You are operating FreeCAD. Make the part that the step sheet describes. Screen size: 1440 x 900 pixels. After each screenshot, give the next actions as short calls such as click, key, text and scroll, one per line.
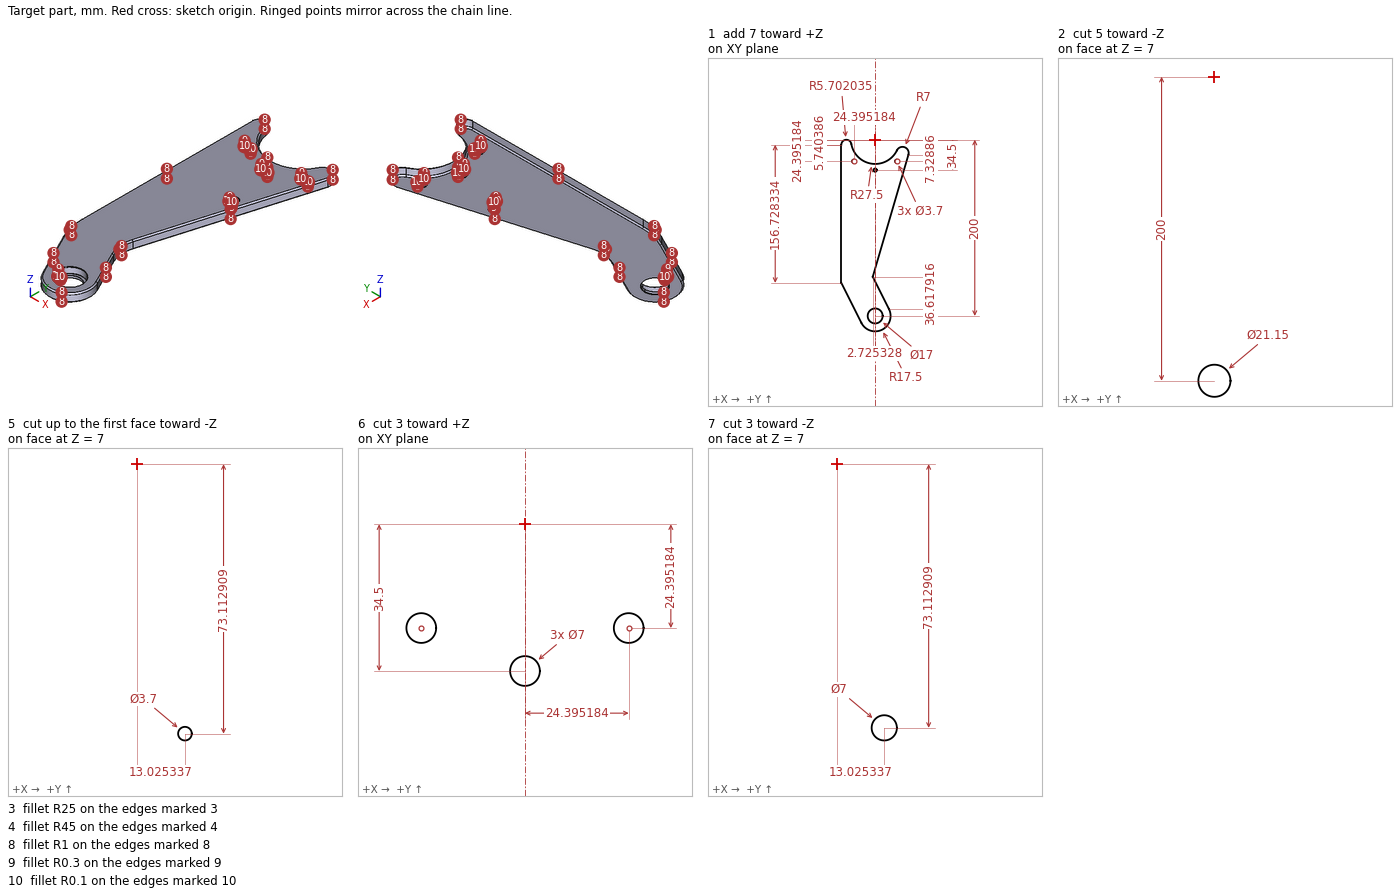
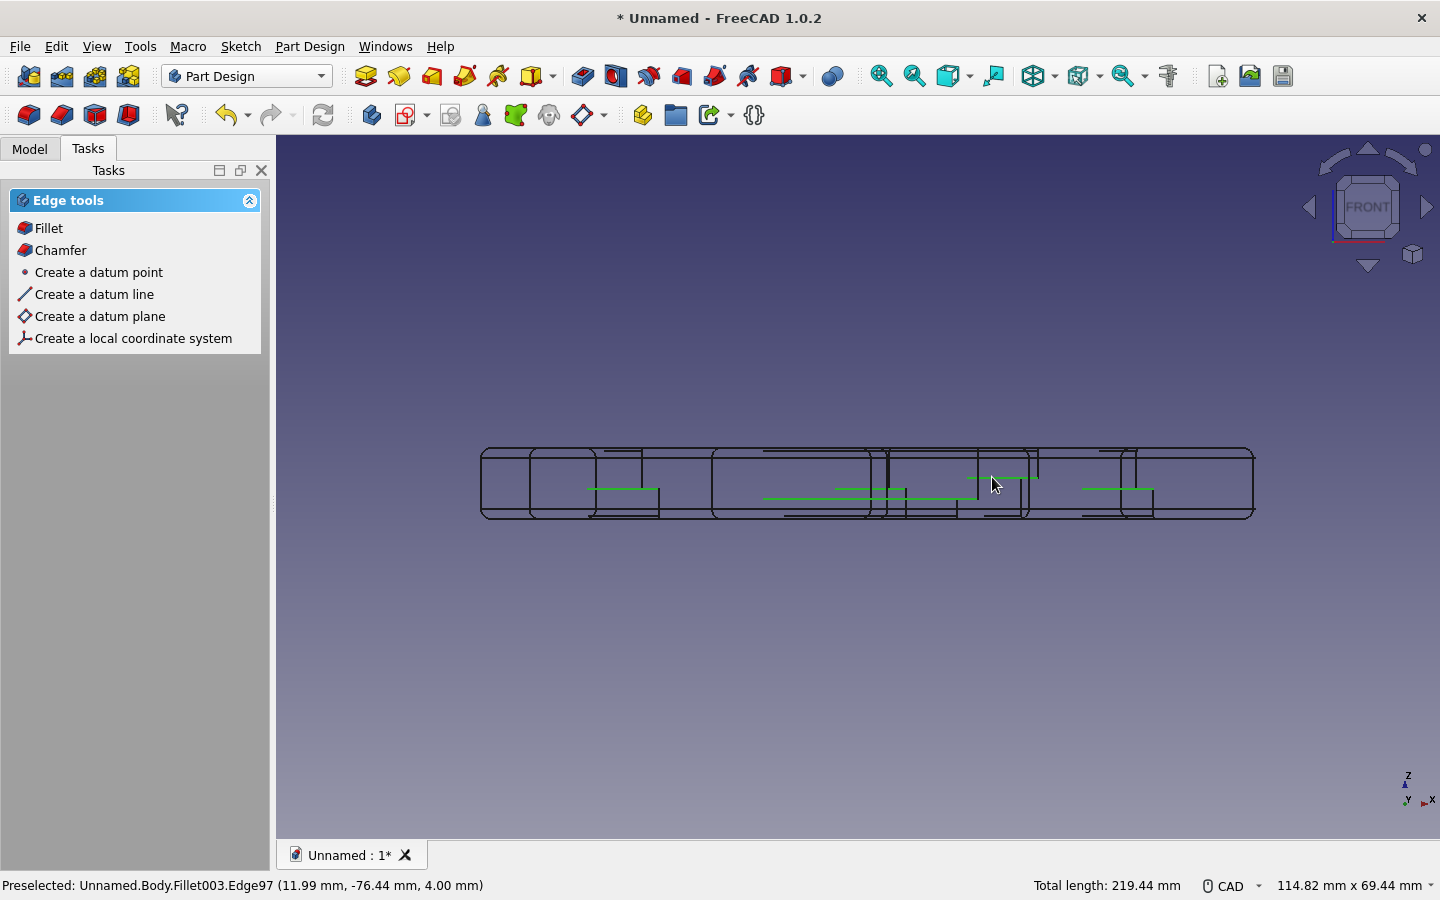
click(882, 76)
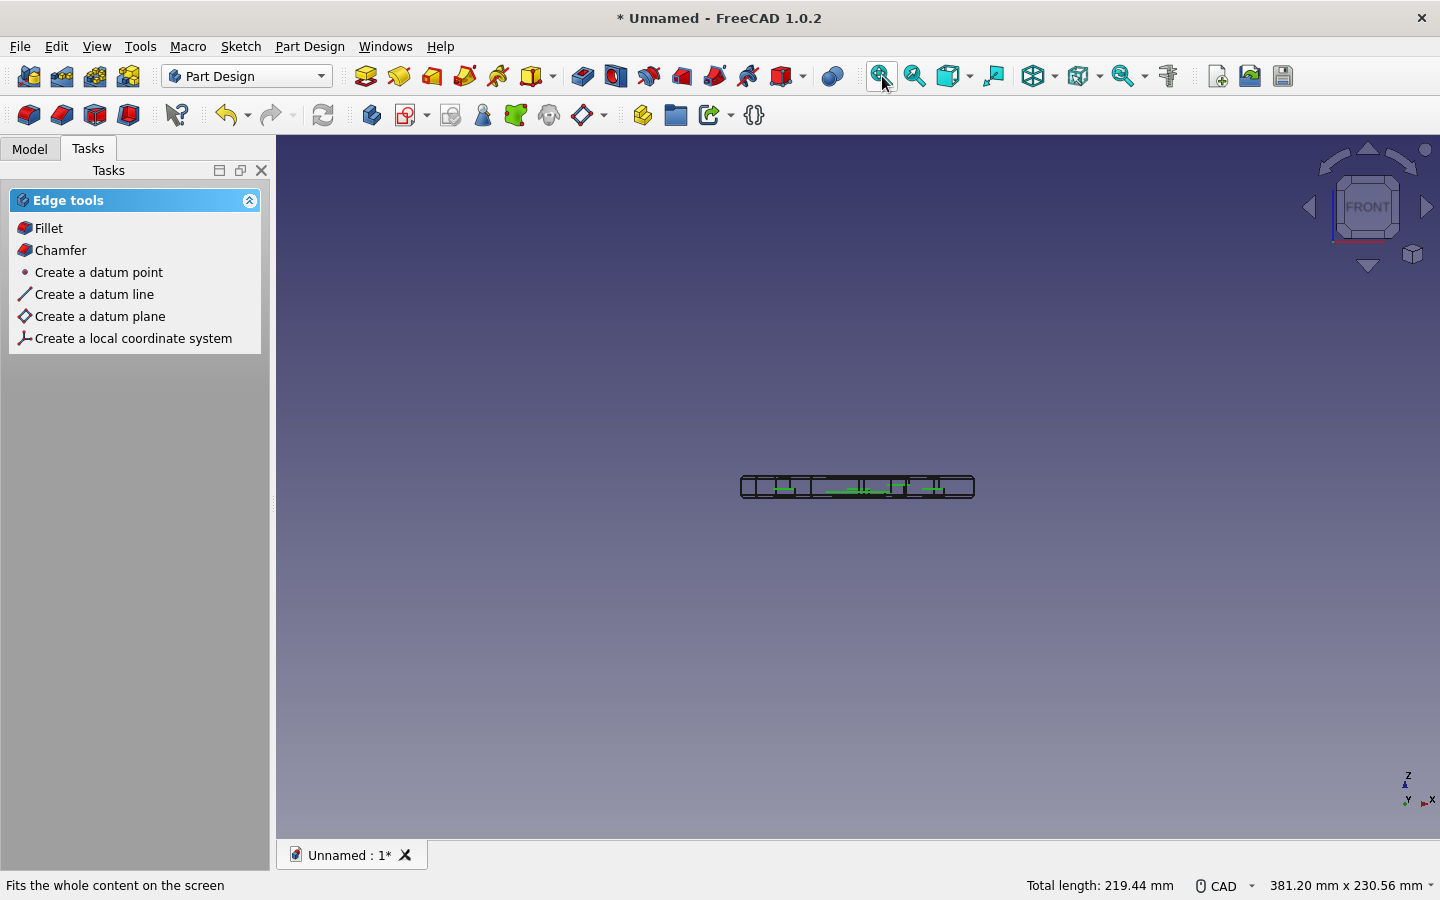
key(3)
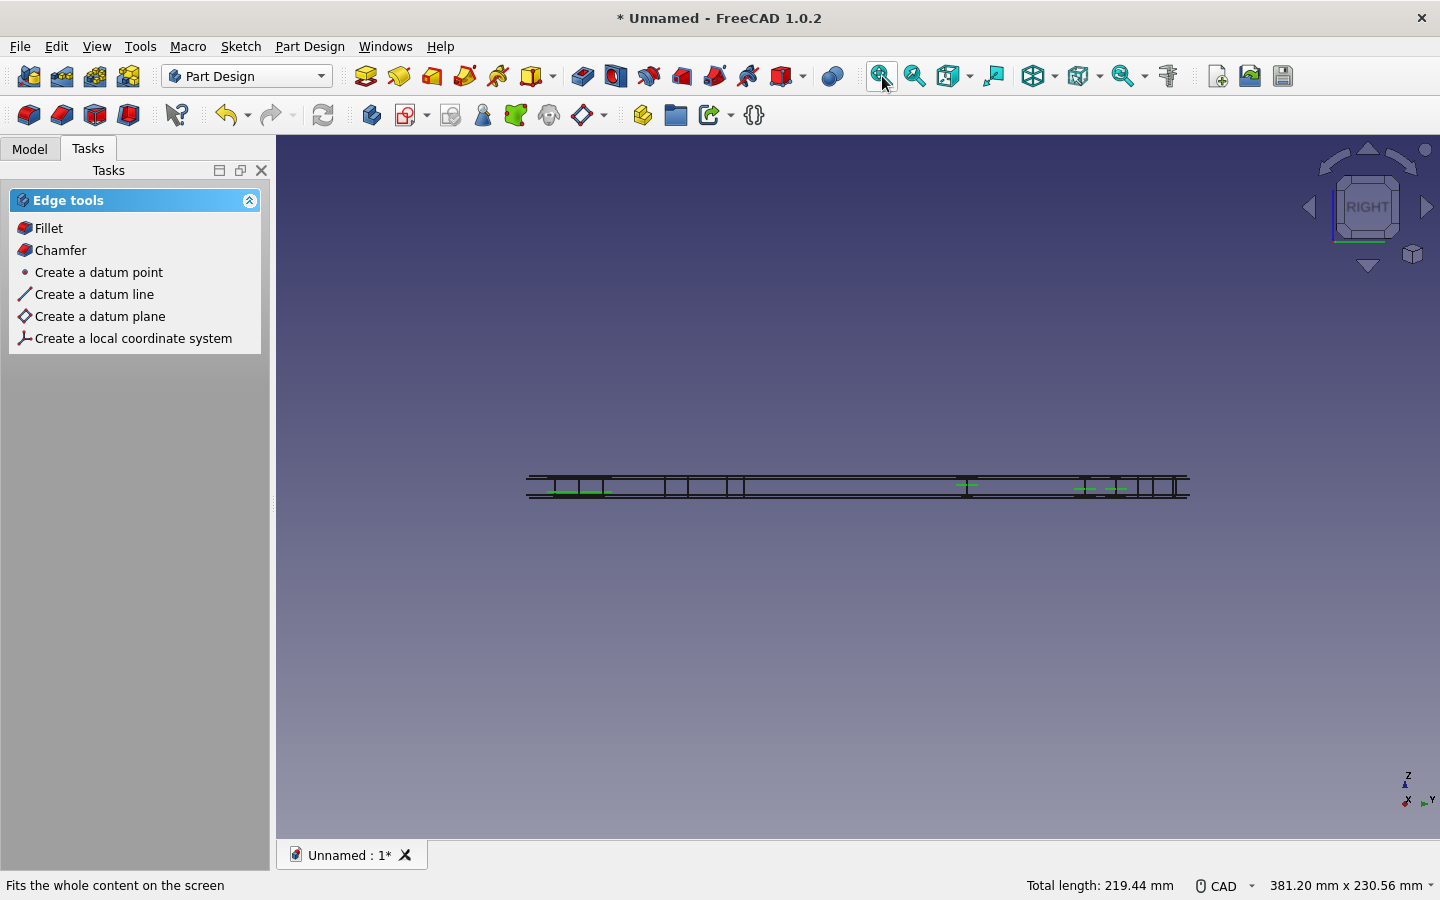
scroll(1085, 488, up, 6)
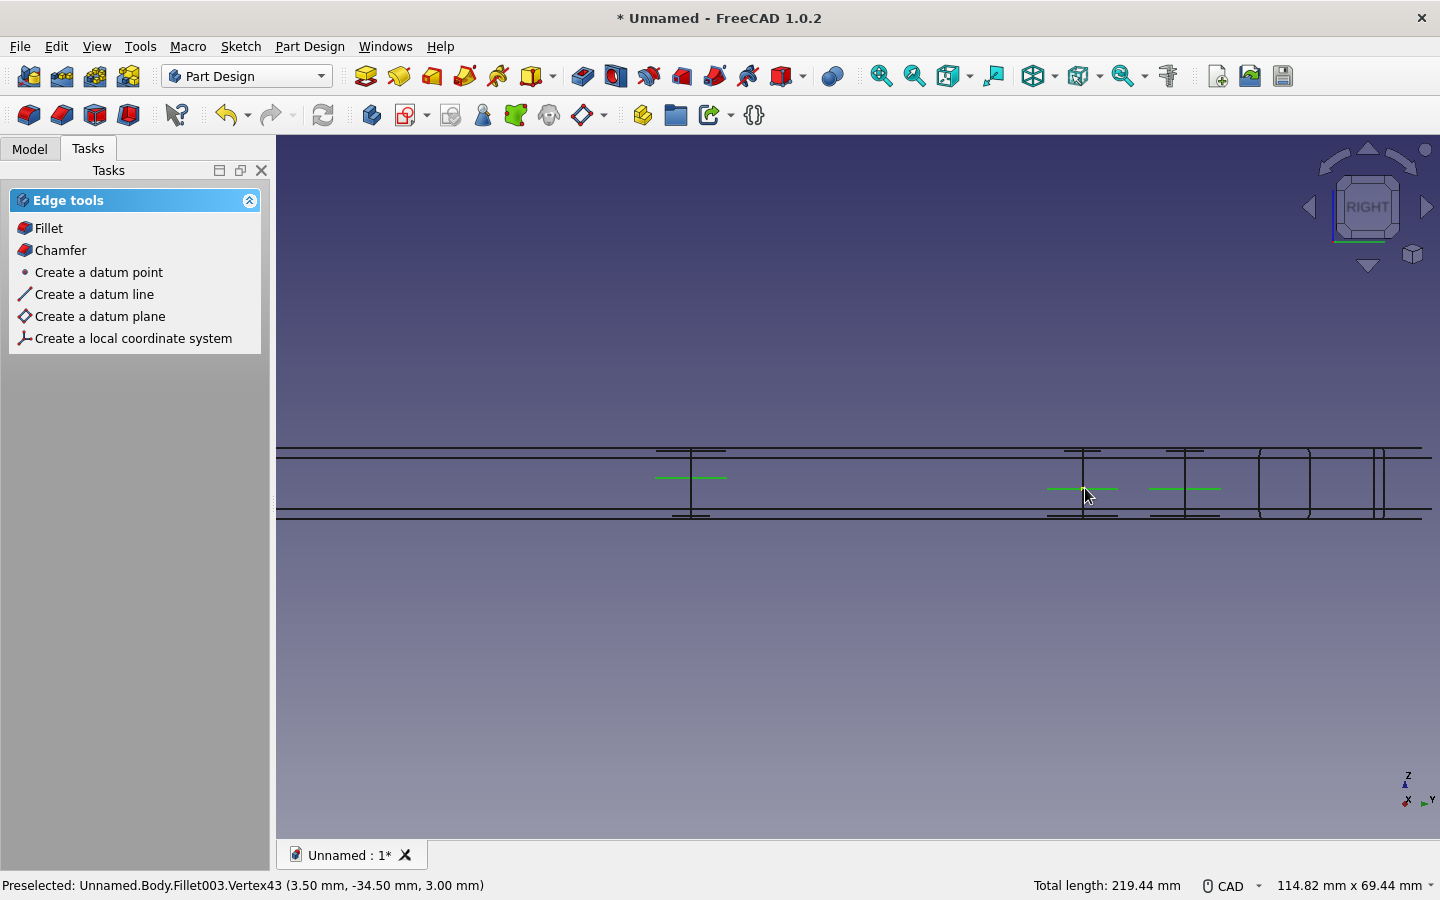
click(882, 76)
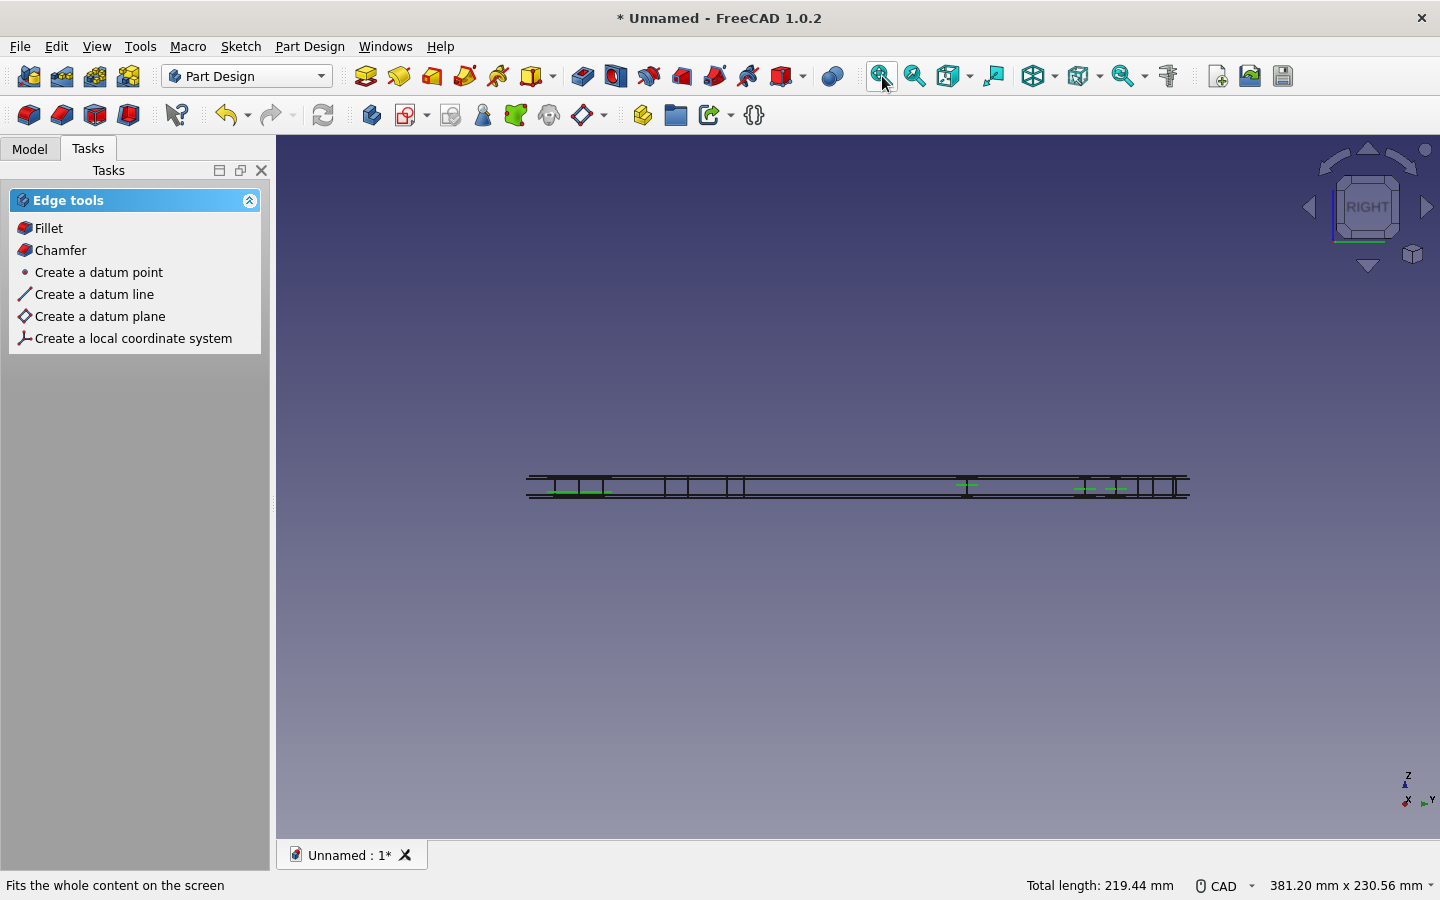
key(5)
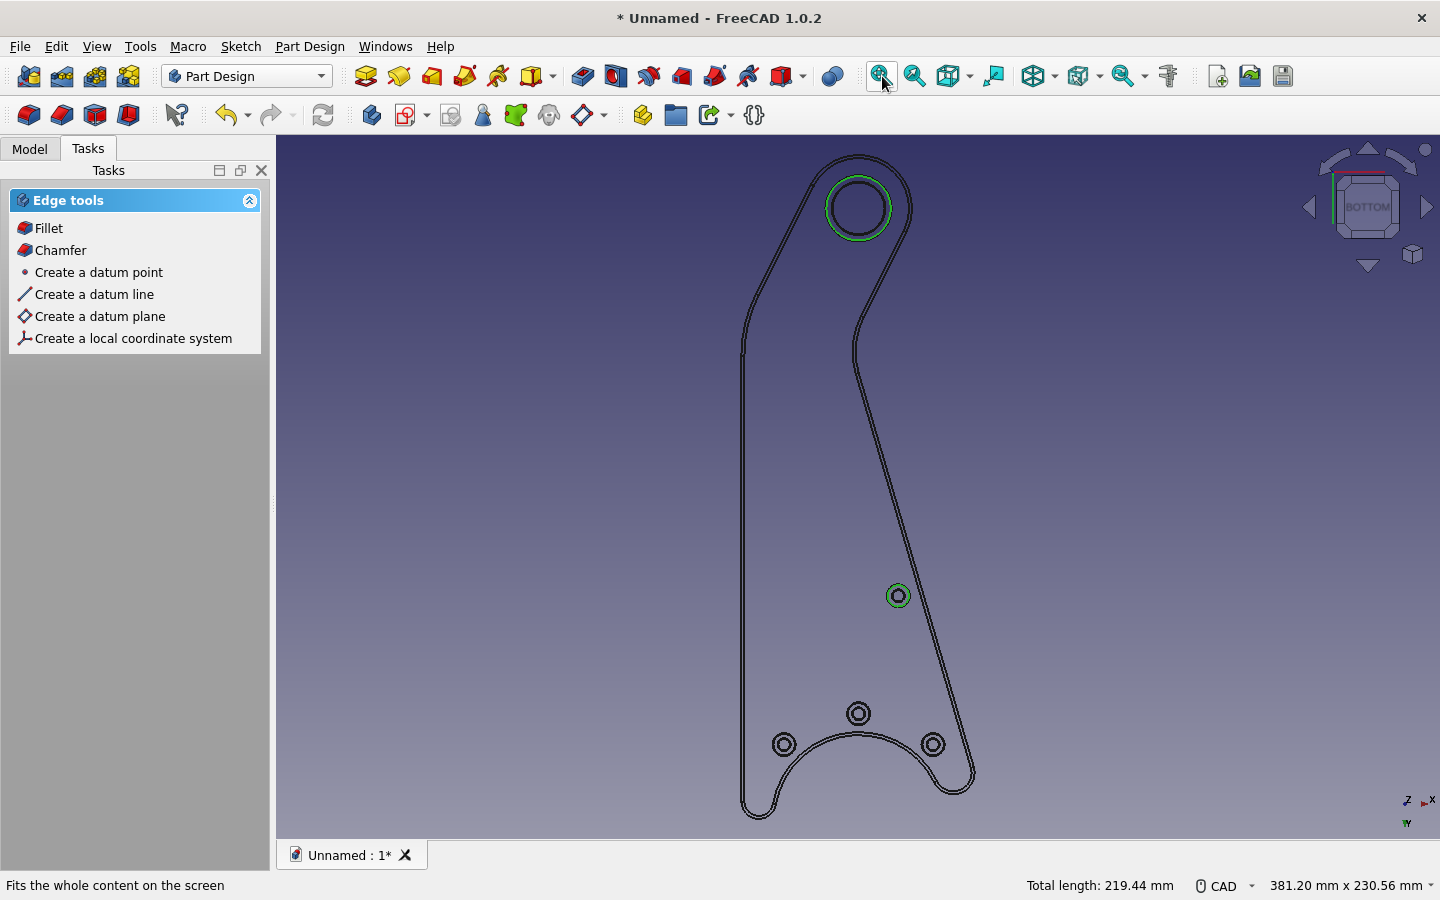
scroll(853, 713, up, 6)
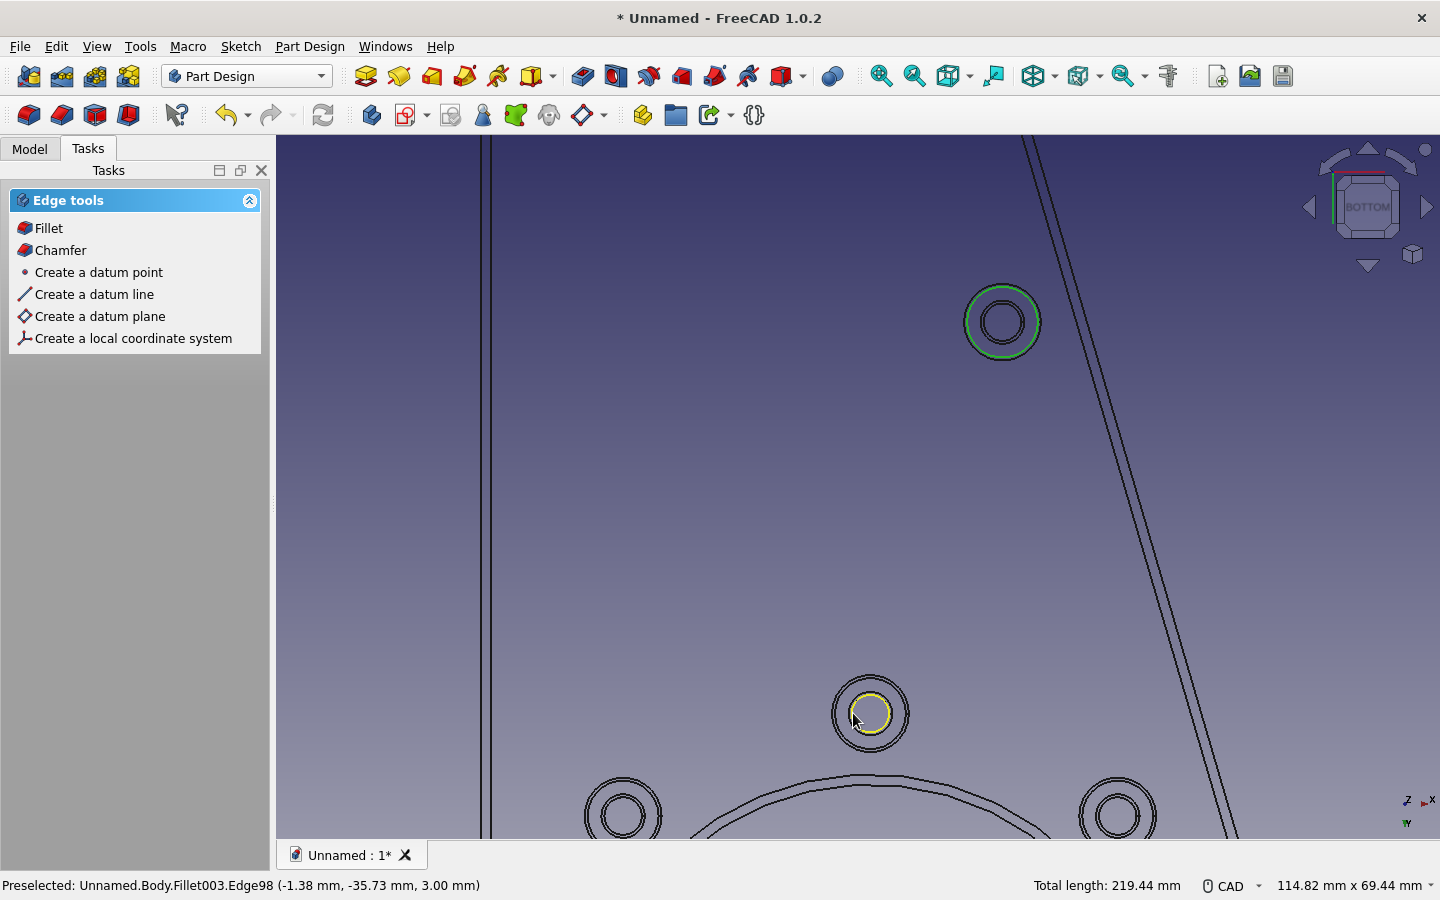
click(852, 713, ctrl)